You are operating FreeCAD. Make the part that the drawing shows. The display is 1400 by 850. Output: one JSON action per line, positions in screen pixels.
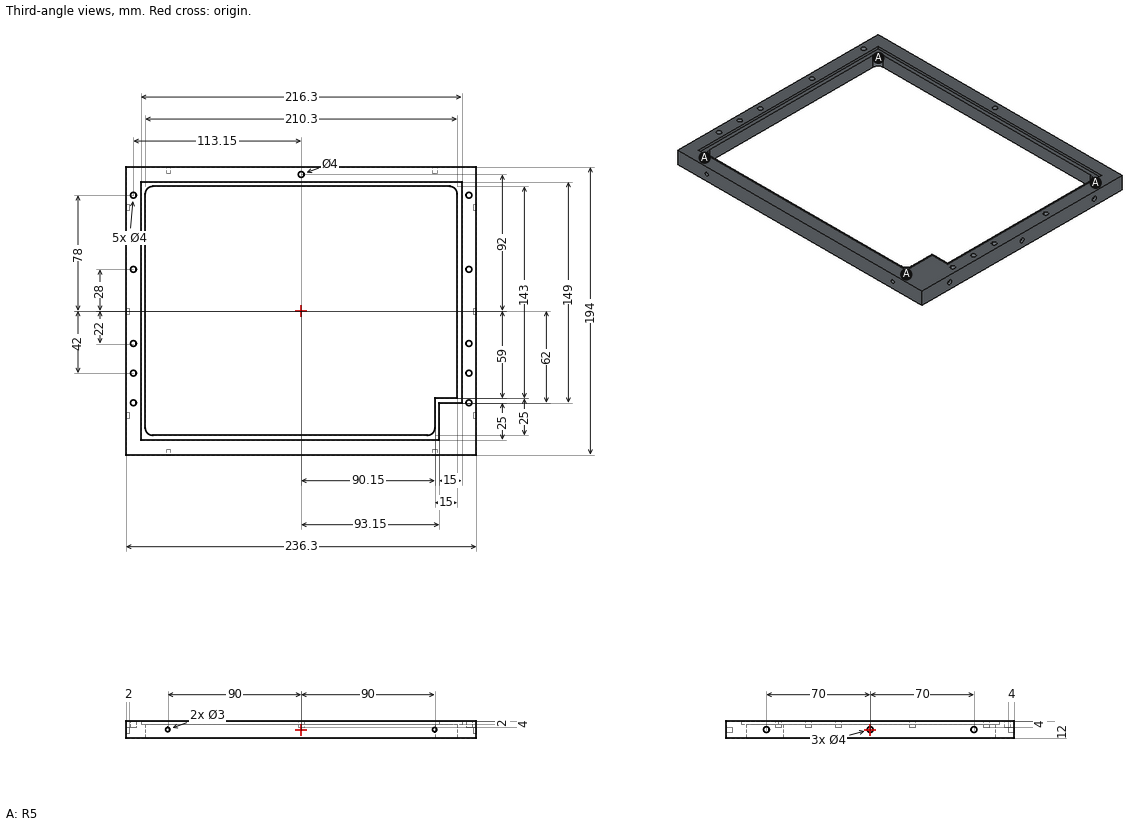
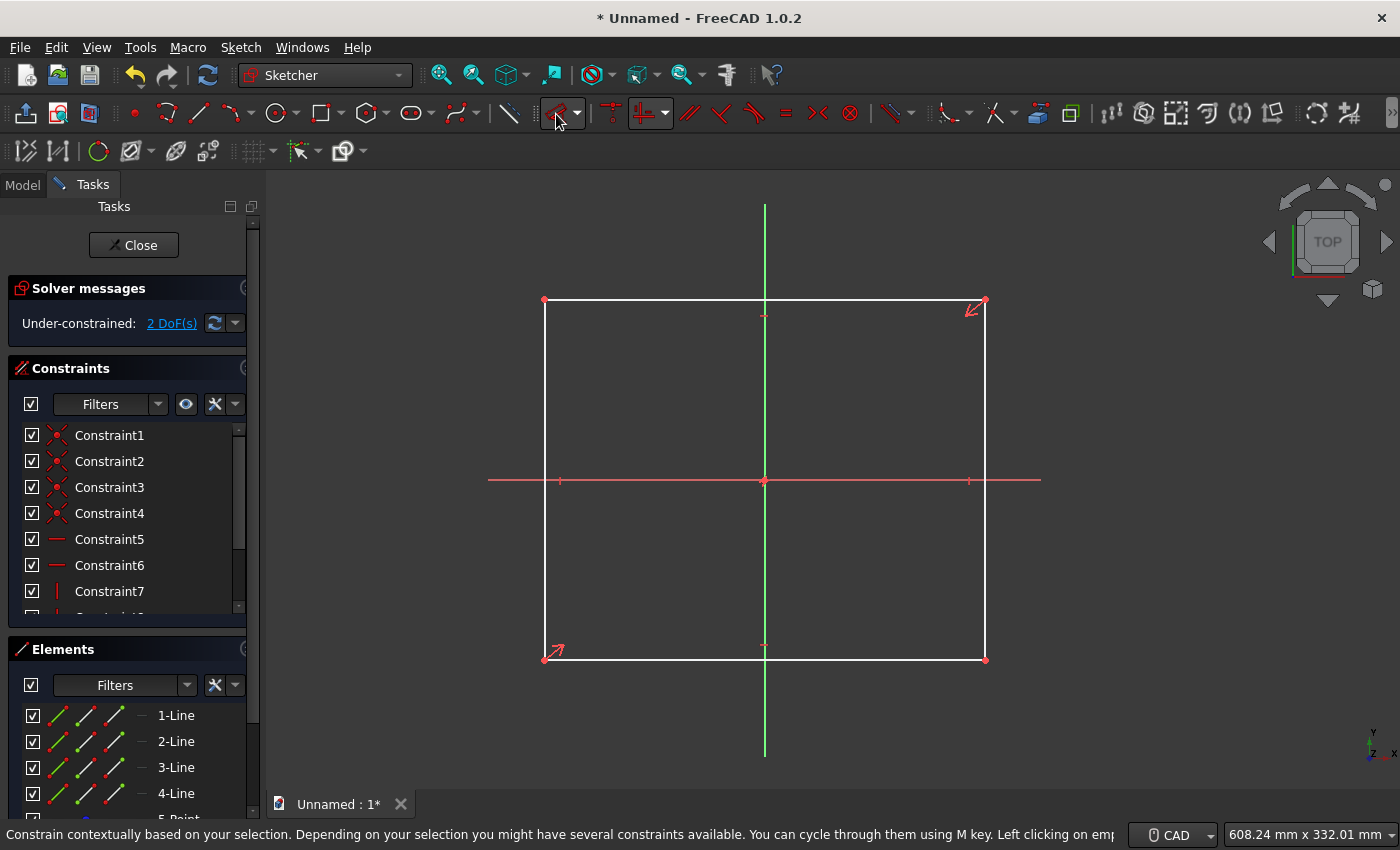
{"action": "left_click", "coordinate": [985, 552]}
{"action": "left_click", "coordinate": [1019, 397]}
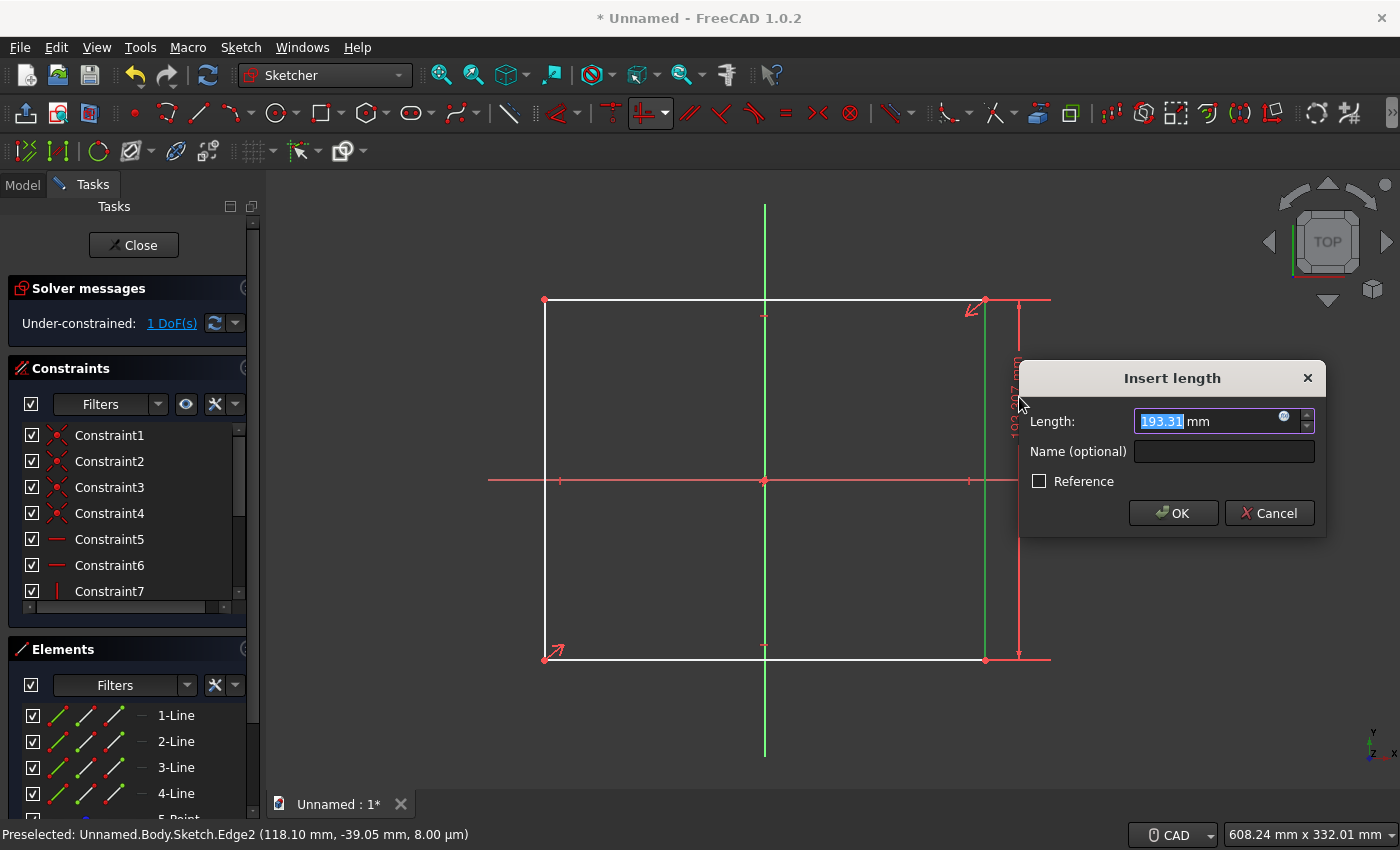
{"action": "type", "text": "194"}
{"action": "key", "text": "Return"}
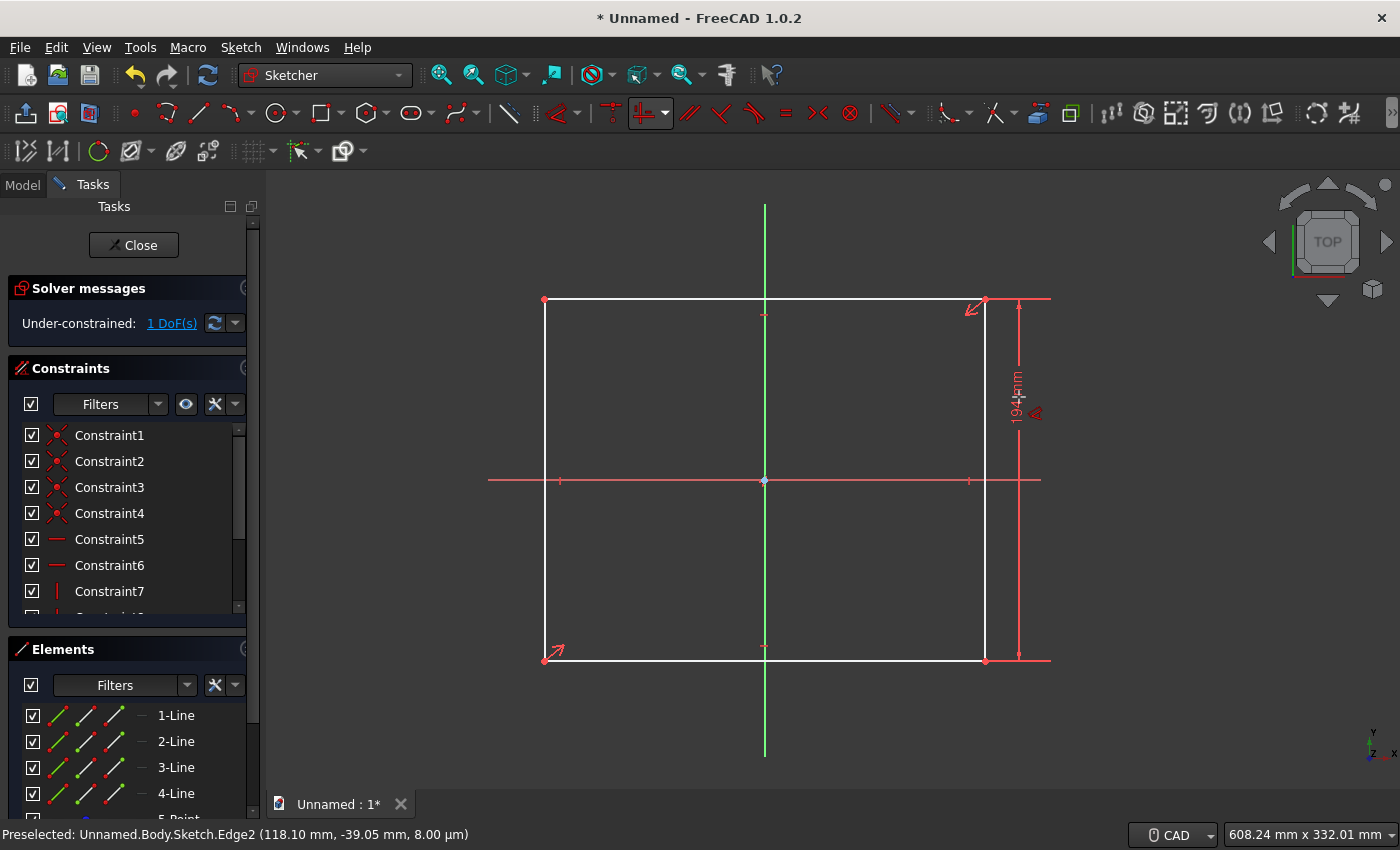
{"action": "left_click", "coordinate": [677, 661]}
{"action": "left_click", "coordinate": [664, 695]}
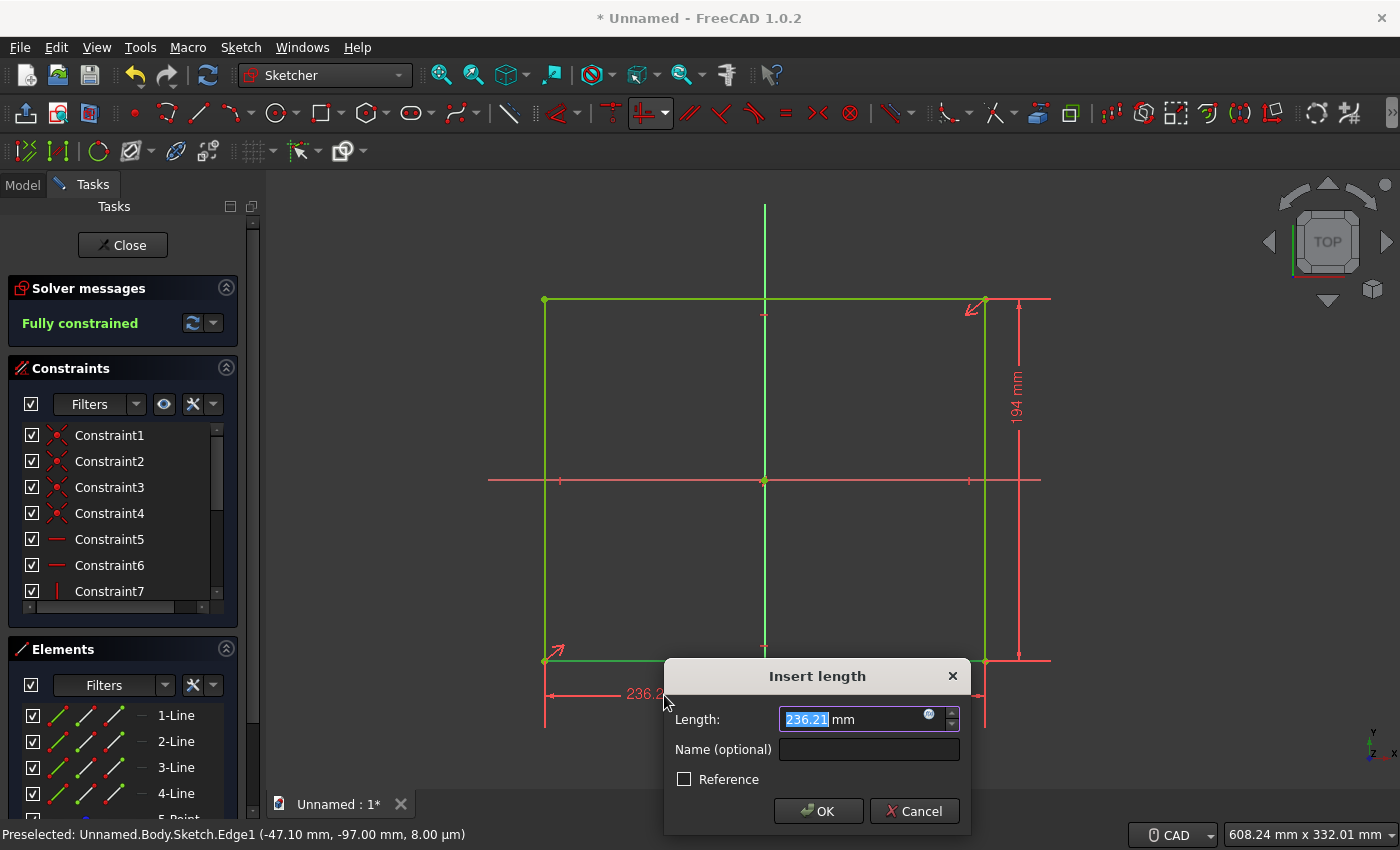
{"action": "type", "text": "236.3"}
{"action": "key", "text": "Return"}
{"action": "key", "text": "Escape"}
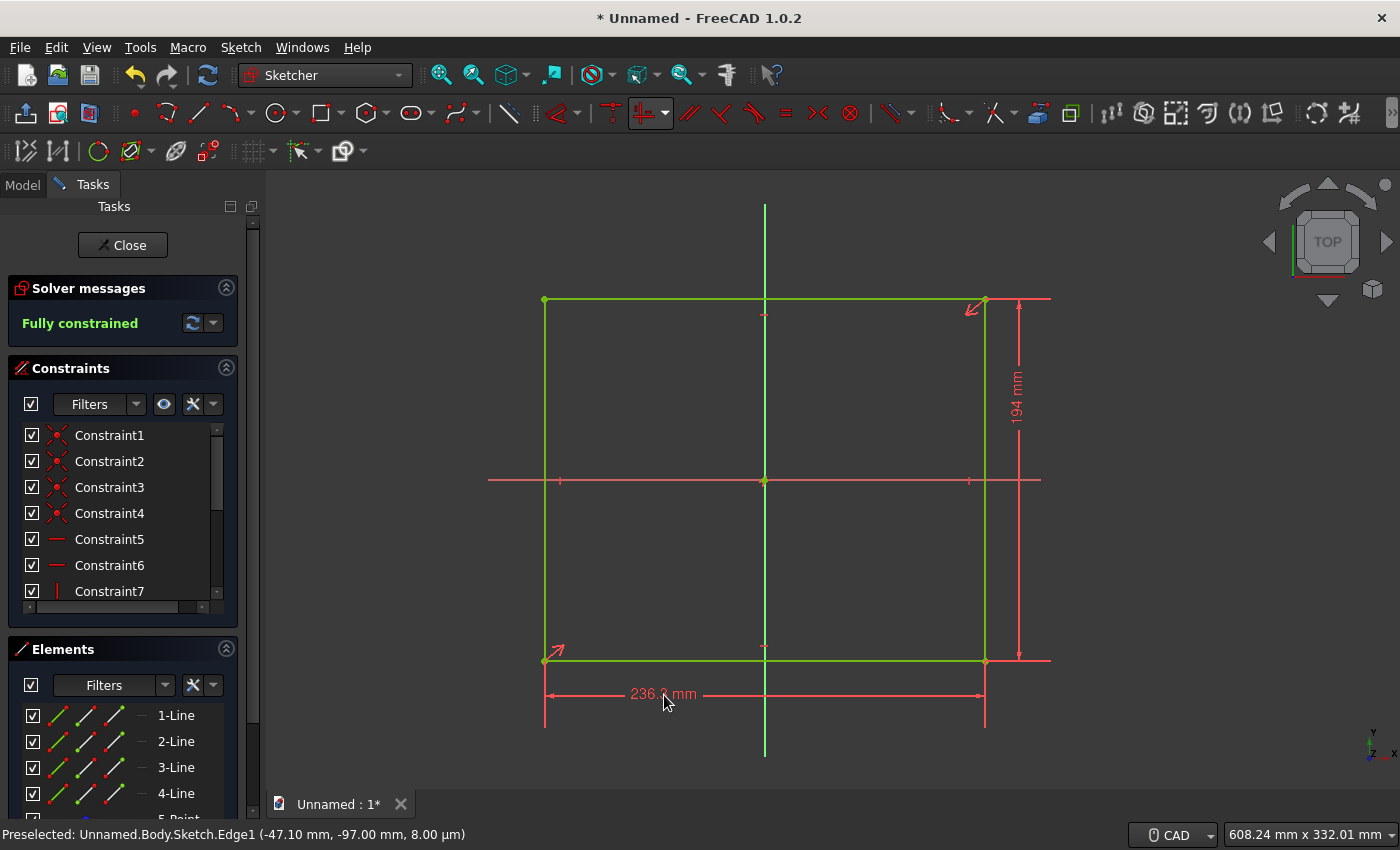
{"action": "left_click", "coordinate": [123, 245]}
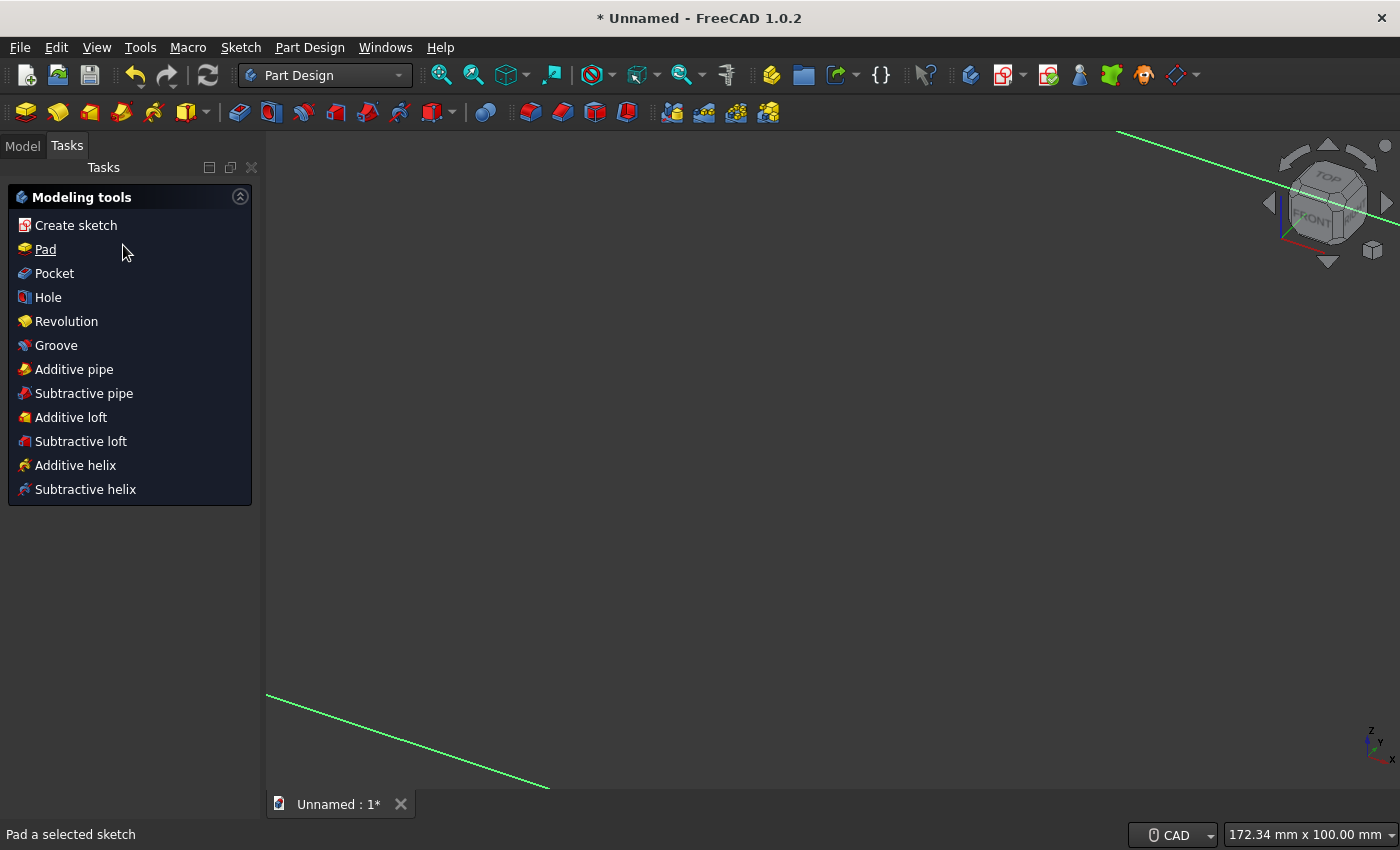
{"action": "left_click", "coordinate": [26, 112]}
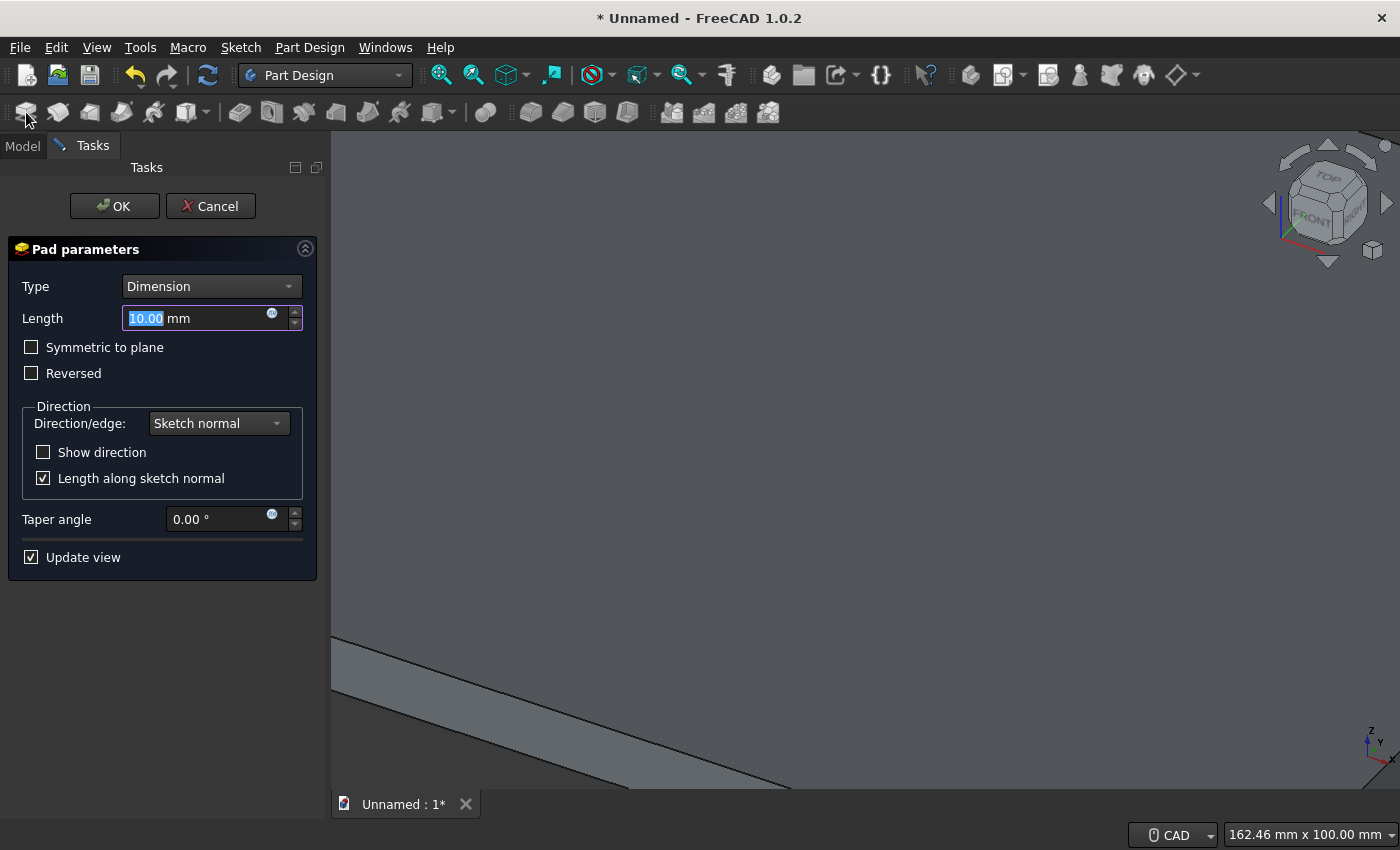
{"action": "type", "text": "12"}
{"action": "key", "text": "Tab"}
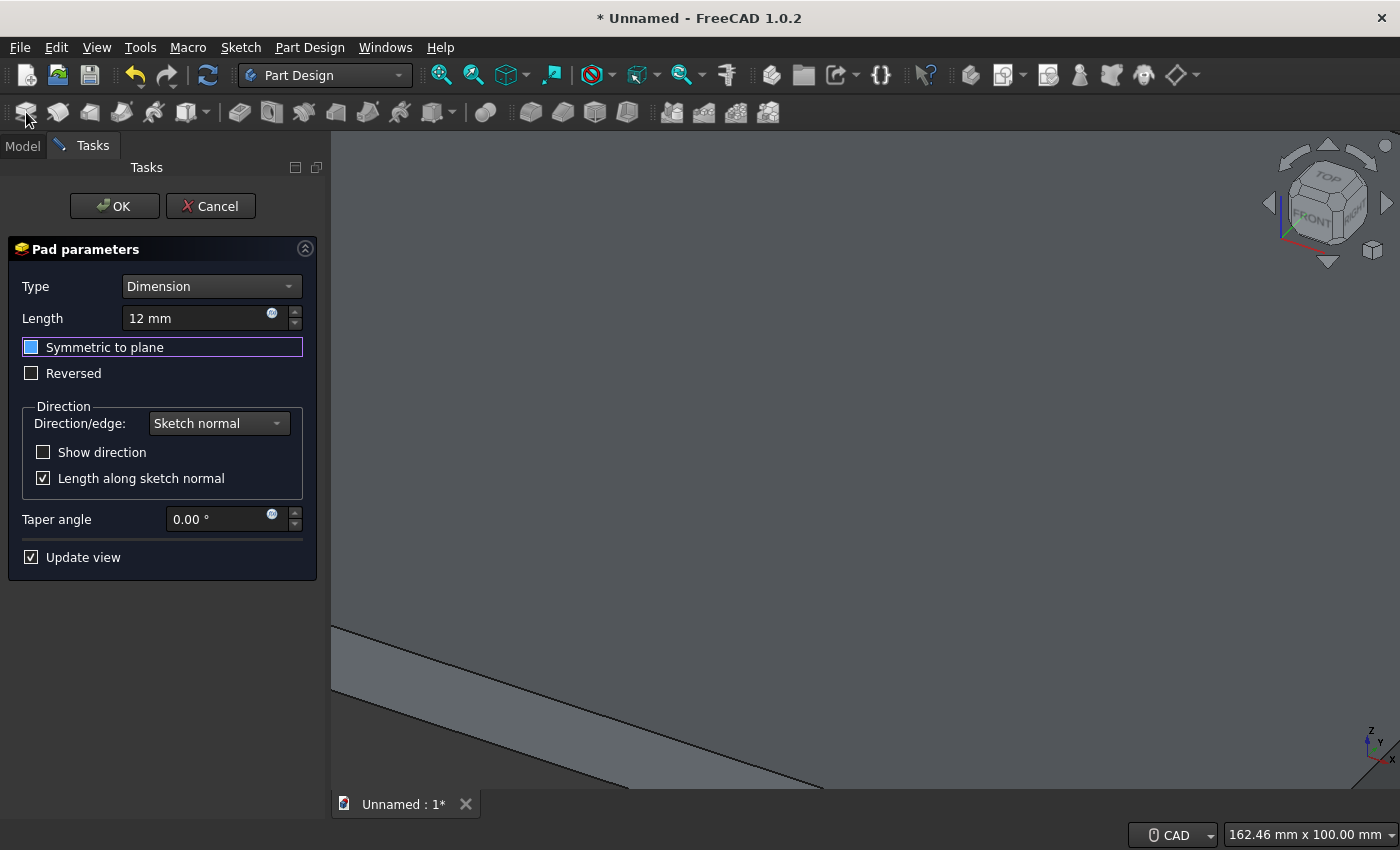
{"action": "left_click", "coordinate": [30, 347]}